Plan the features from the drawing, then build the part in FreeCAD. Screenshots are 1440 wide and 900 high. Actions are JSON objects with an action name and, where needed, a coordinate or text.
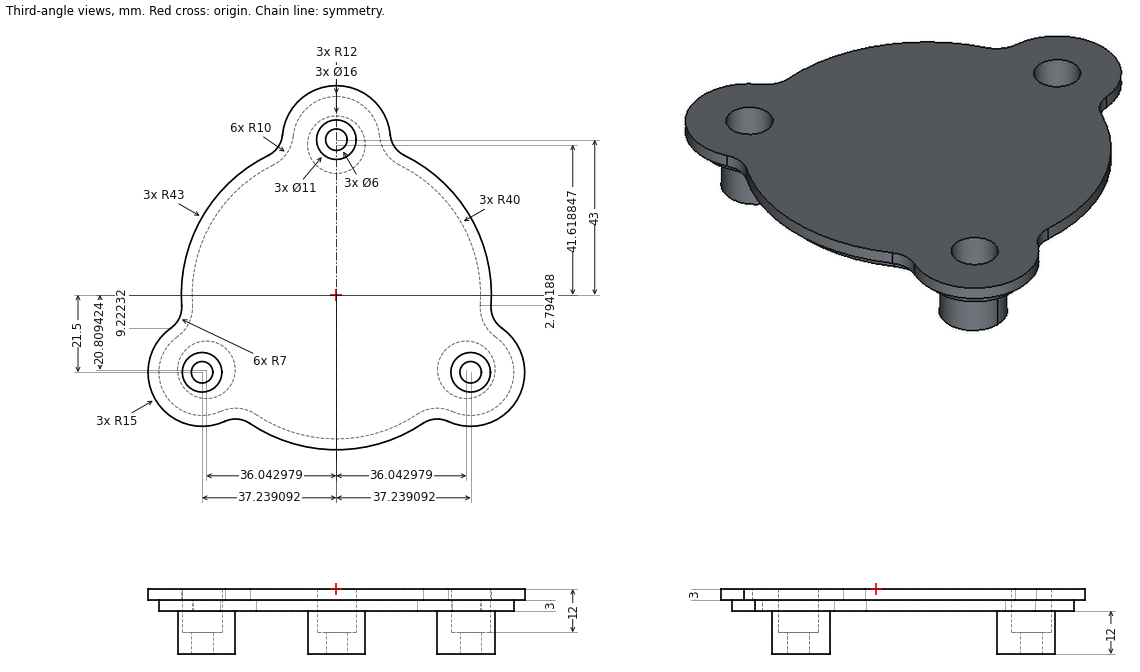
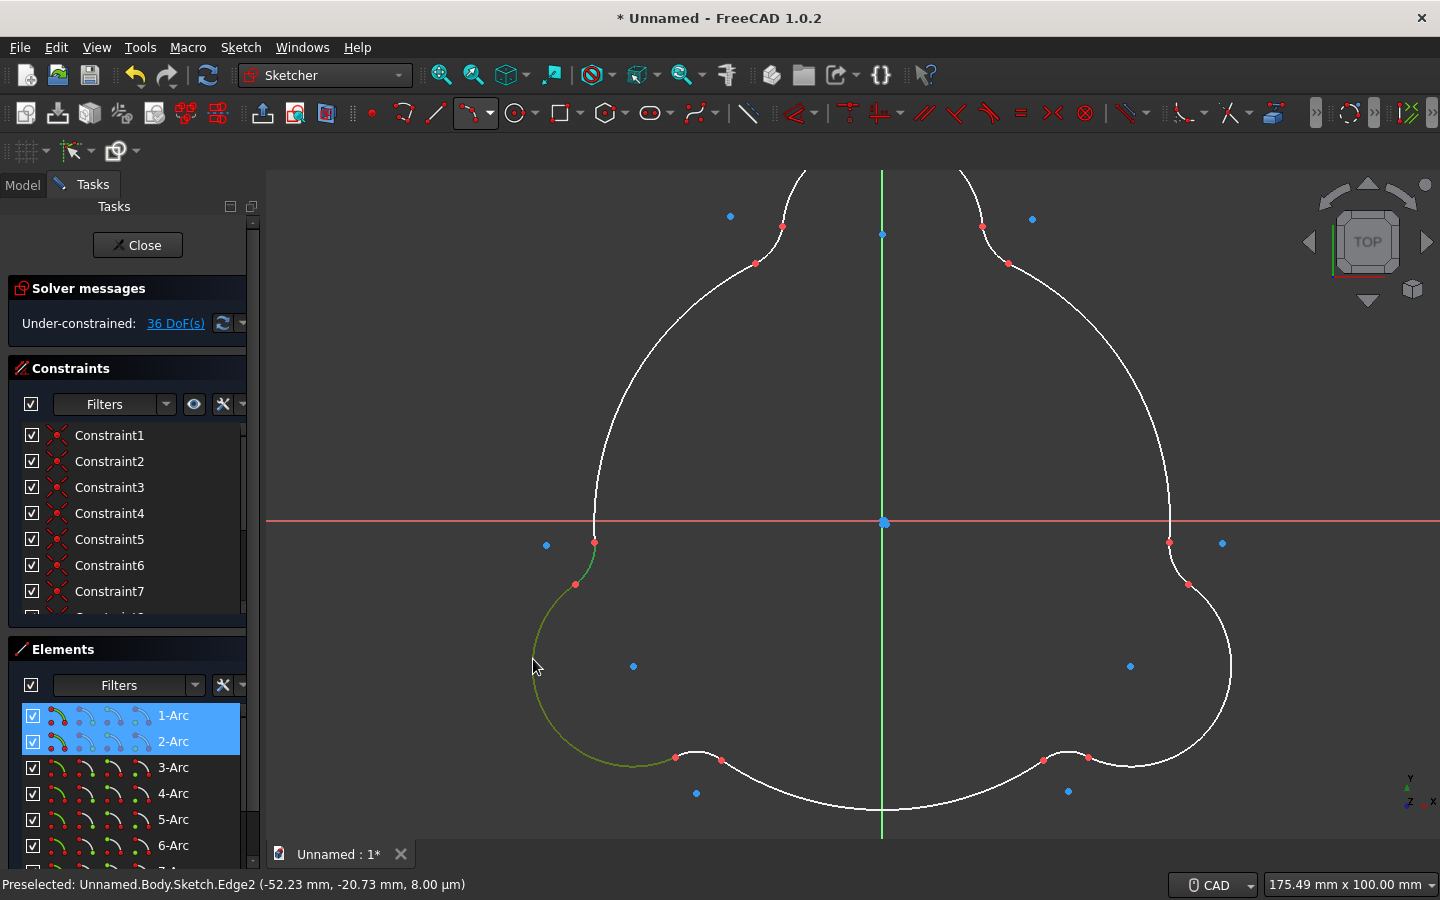
{"action": "left_click", "coordinate": [990, 114]}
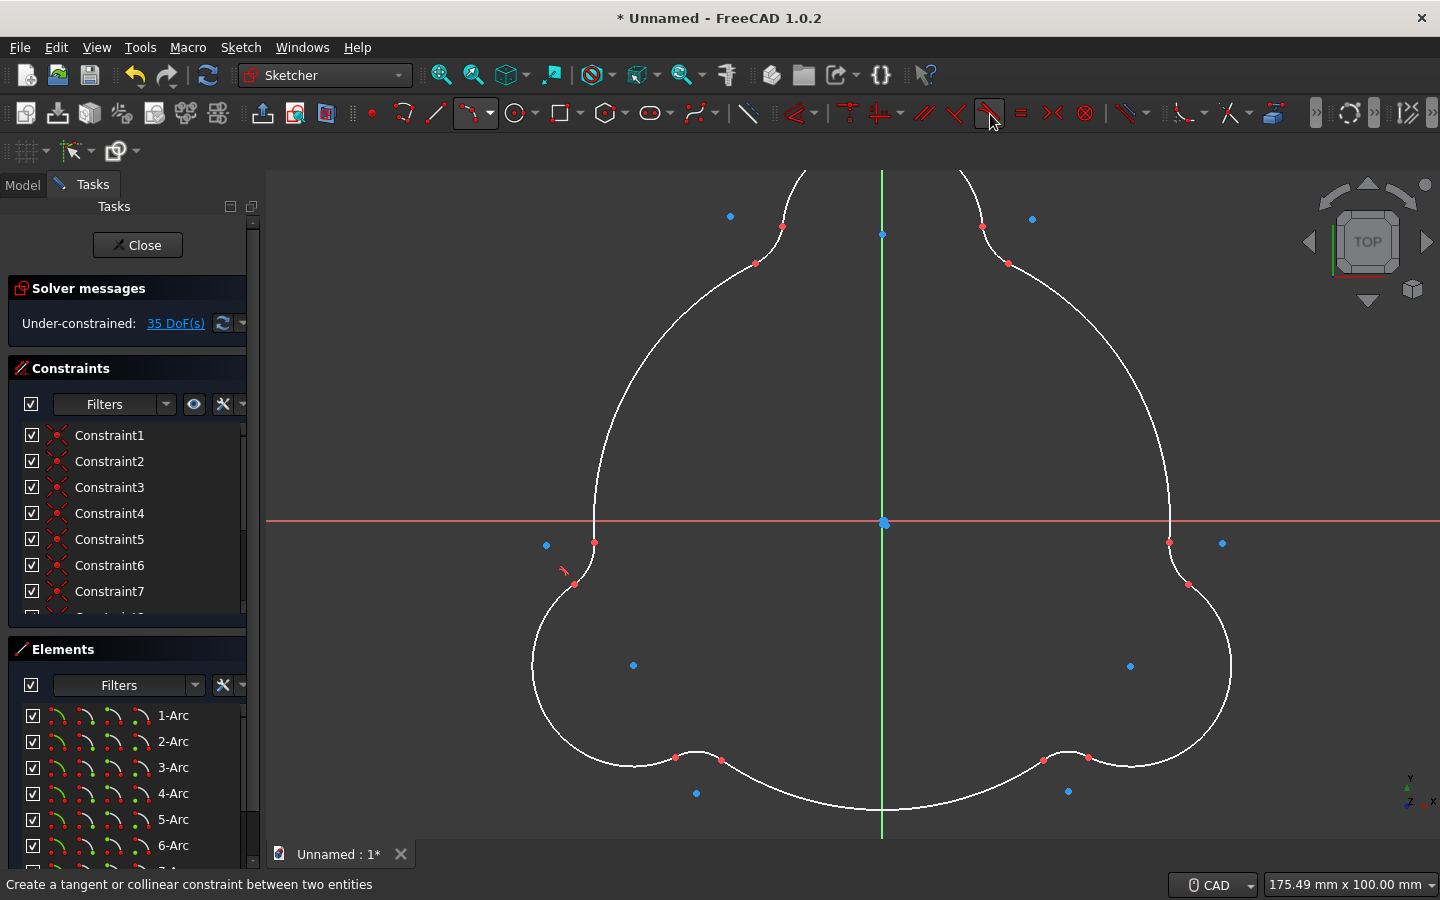
{"action": "left_click", "coordinate": [585, 574]}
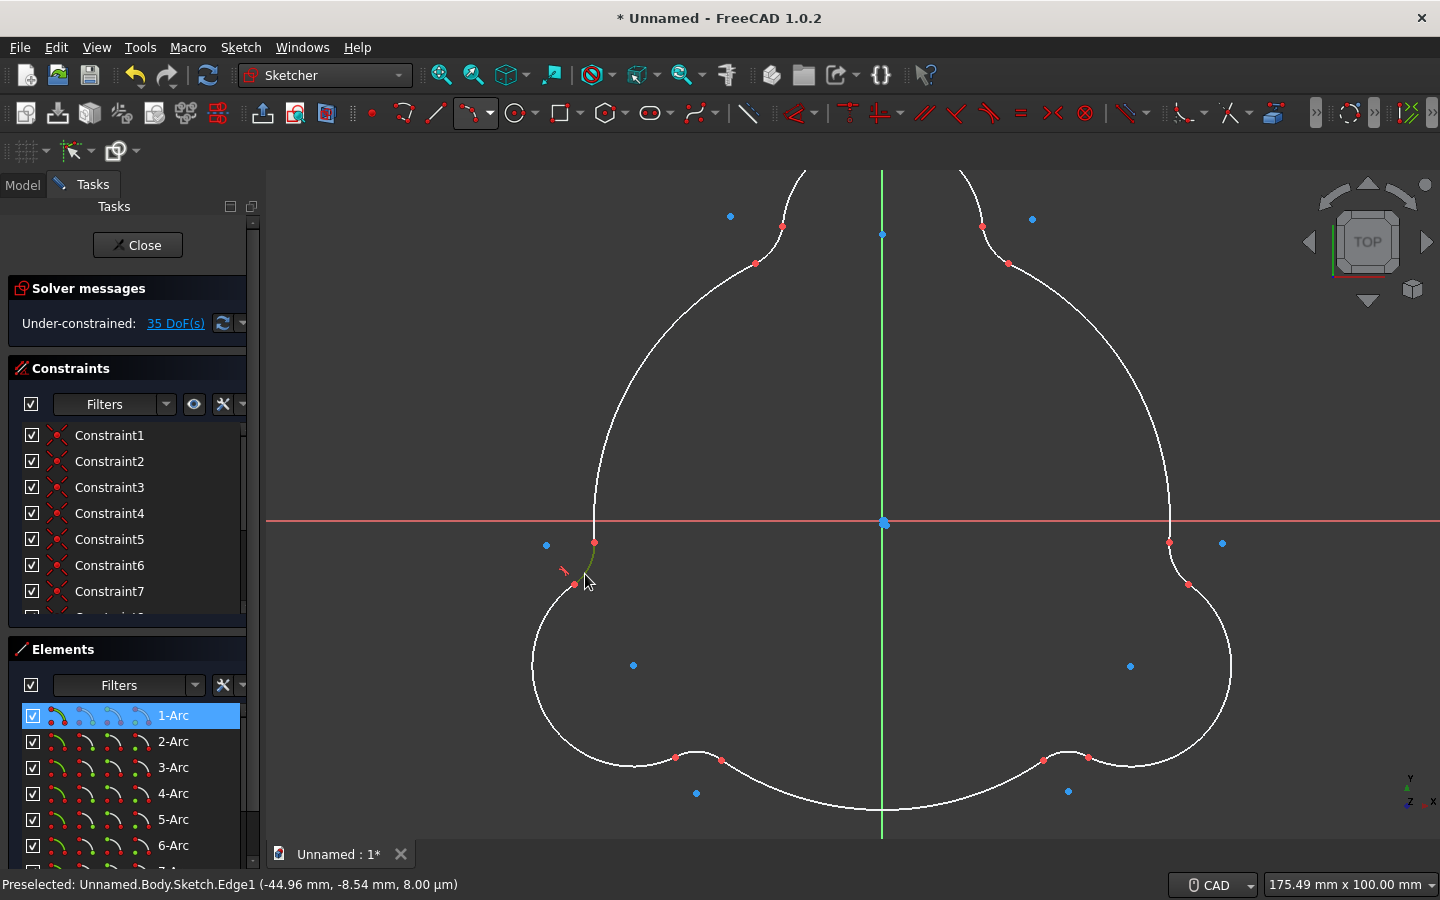
{"action": "left_click", "coordinate": [674, 324]}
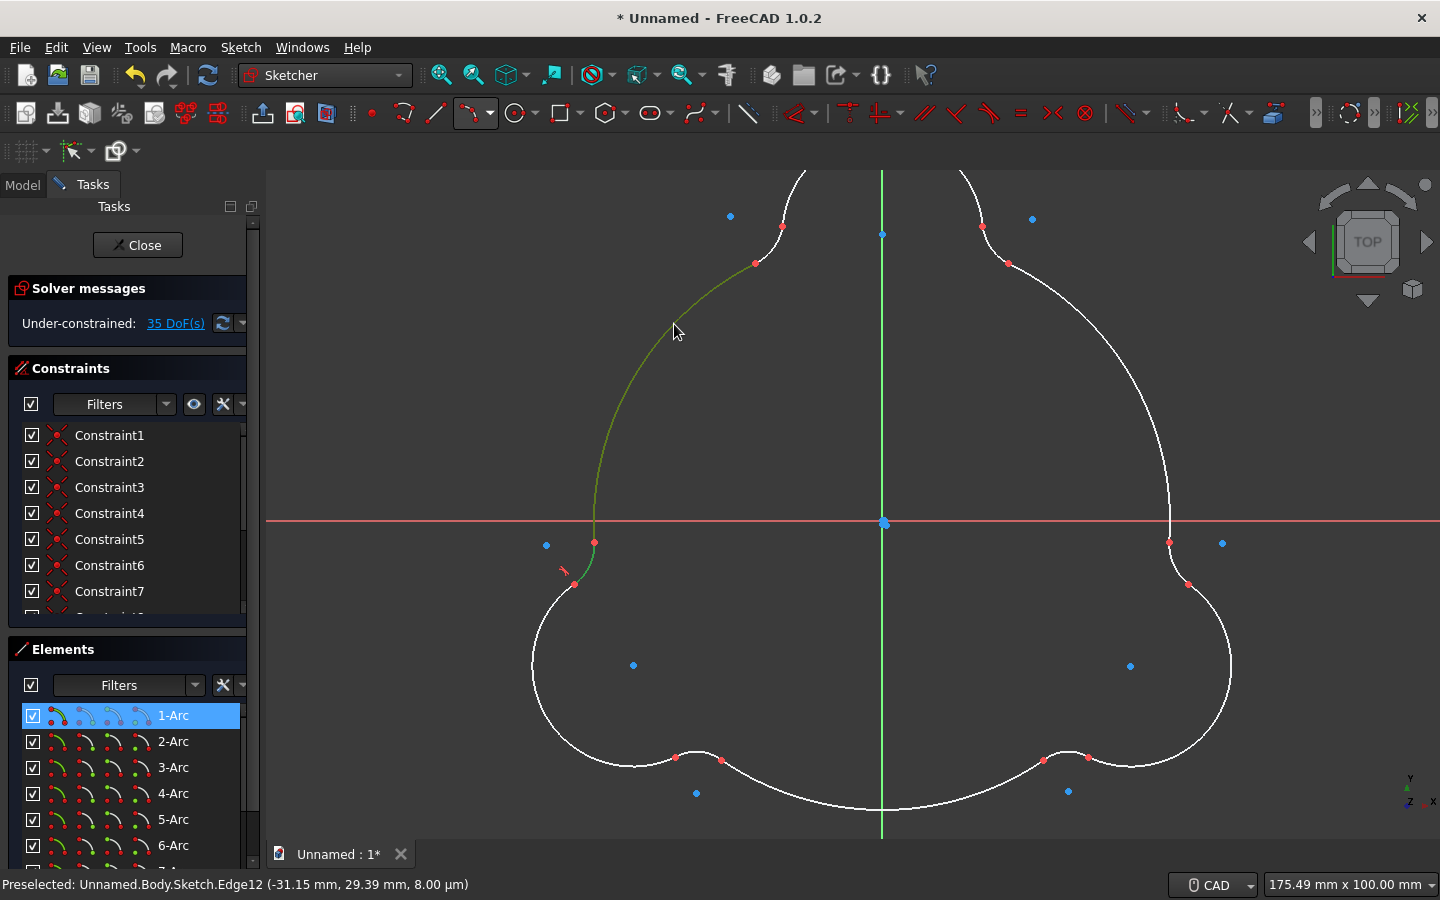
{"action": "left_click", "coordinate": [990, 114]}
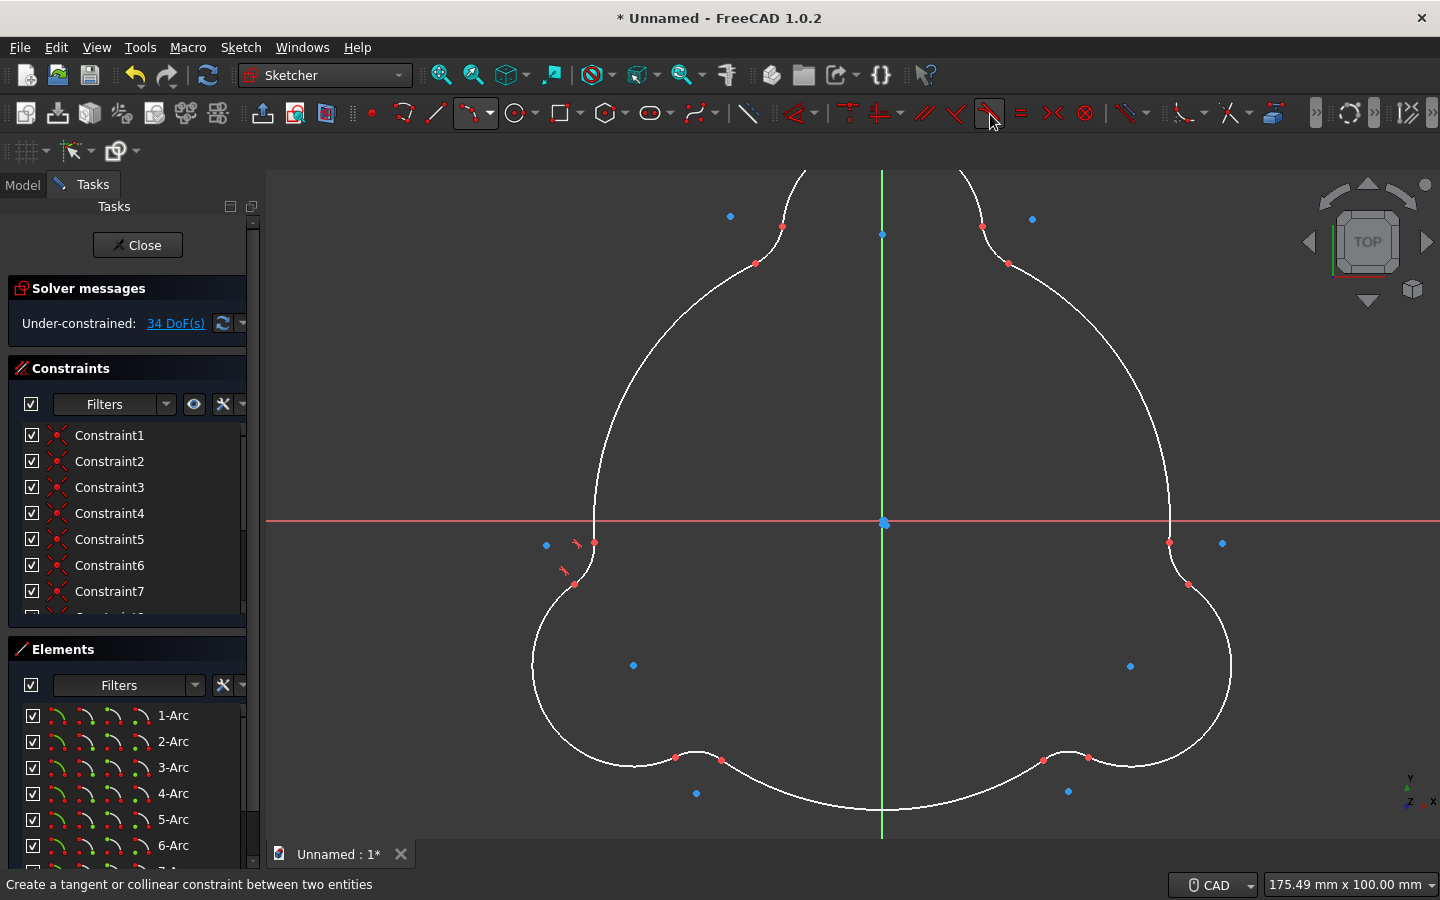
{"action": "left_click", "coordinate": [533, 660]}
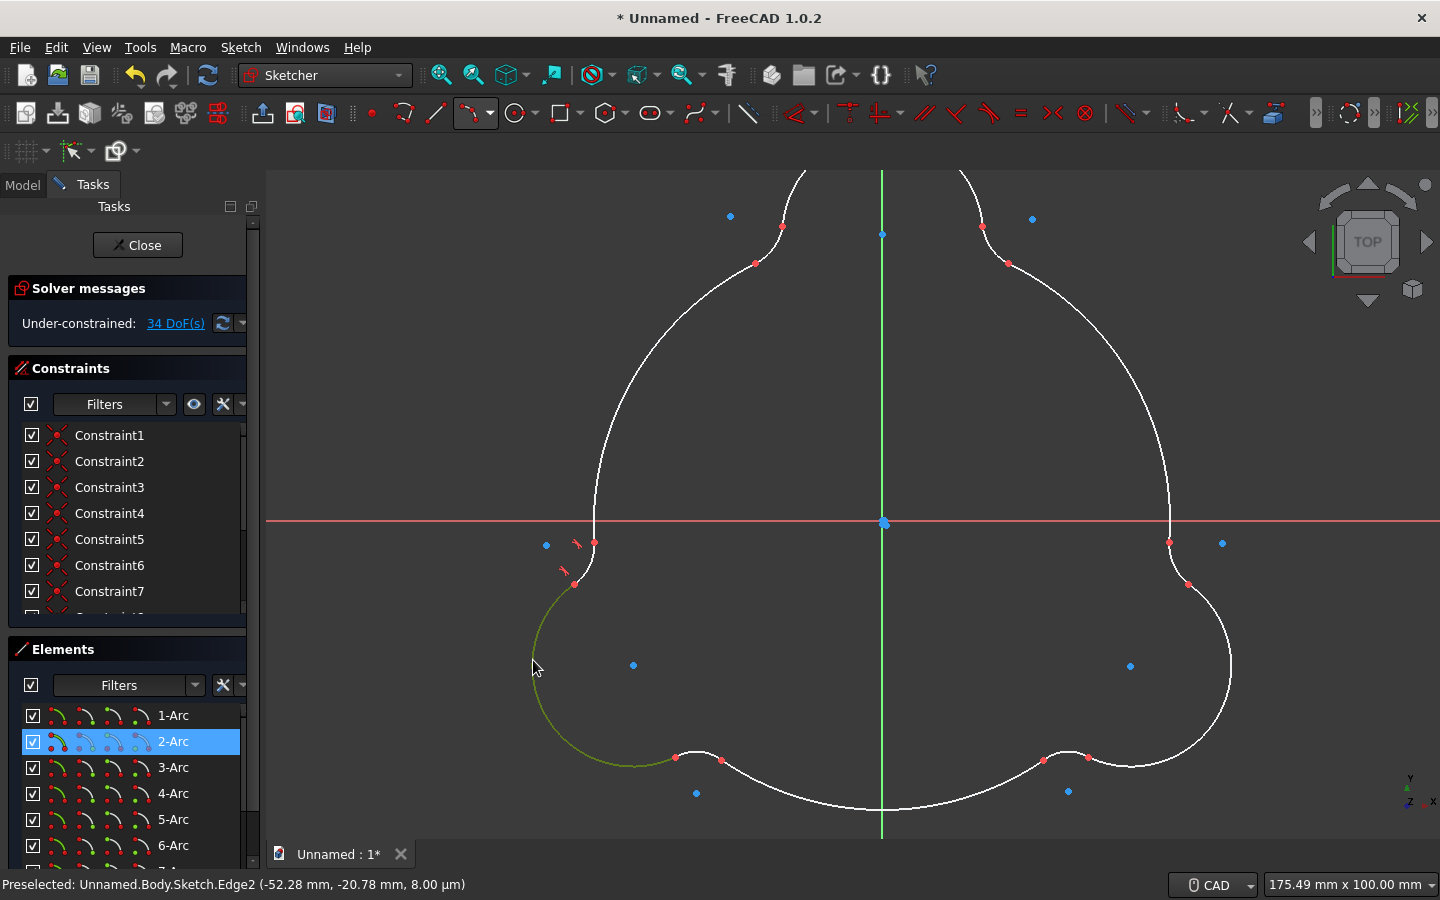
{"action": "left_click", "coordinate": [709, 754]}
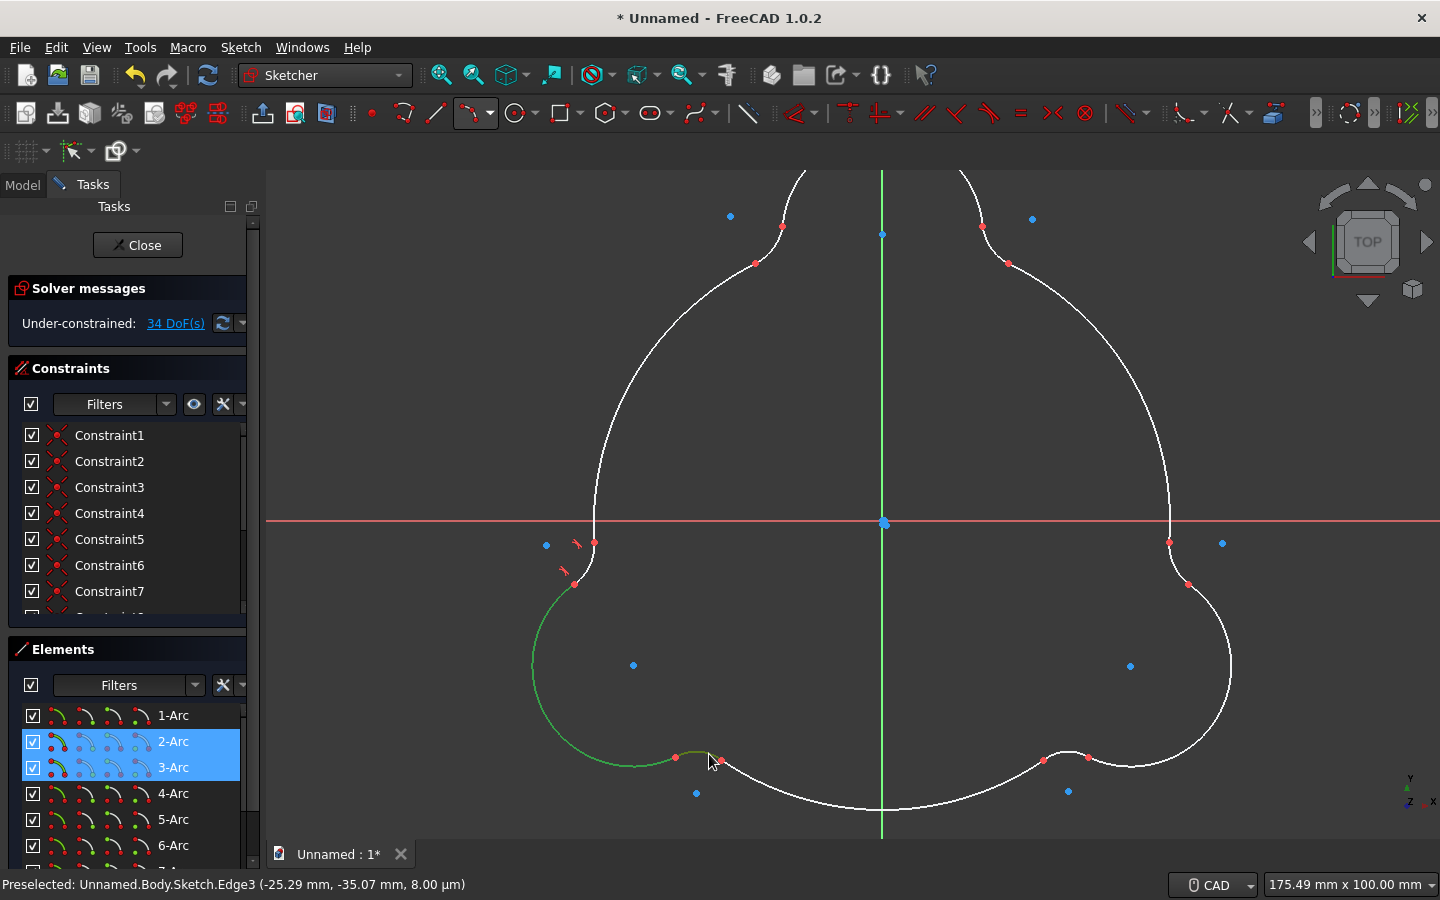
{"action": "left_click", "coordinate": [990, 114]}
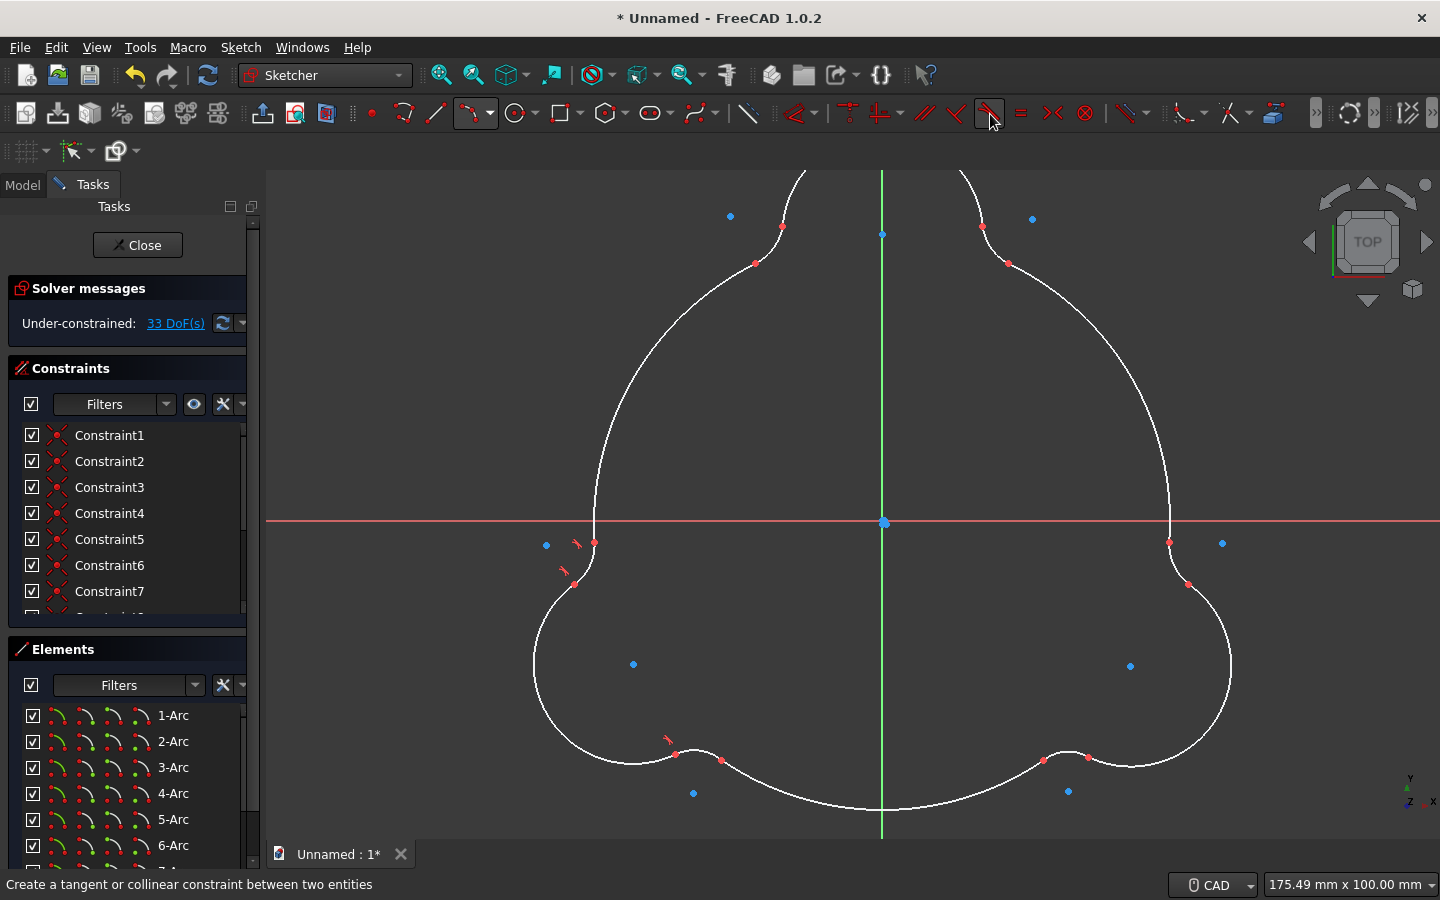
{"action": "left_click", "coordinate": [709, 753]}